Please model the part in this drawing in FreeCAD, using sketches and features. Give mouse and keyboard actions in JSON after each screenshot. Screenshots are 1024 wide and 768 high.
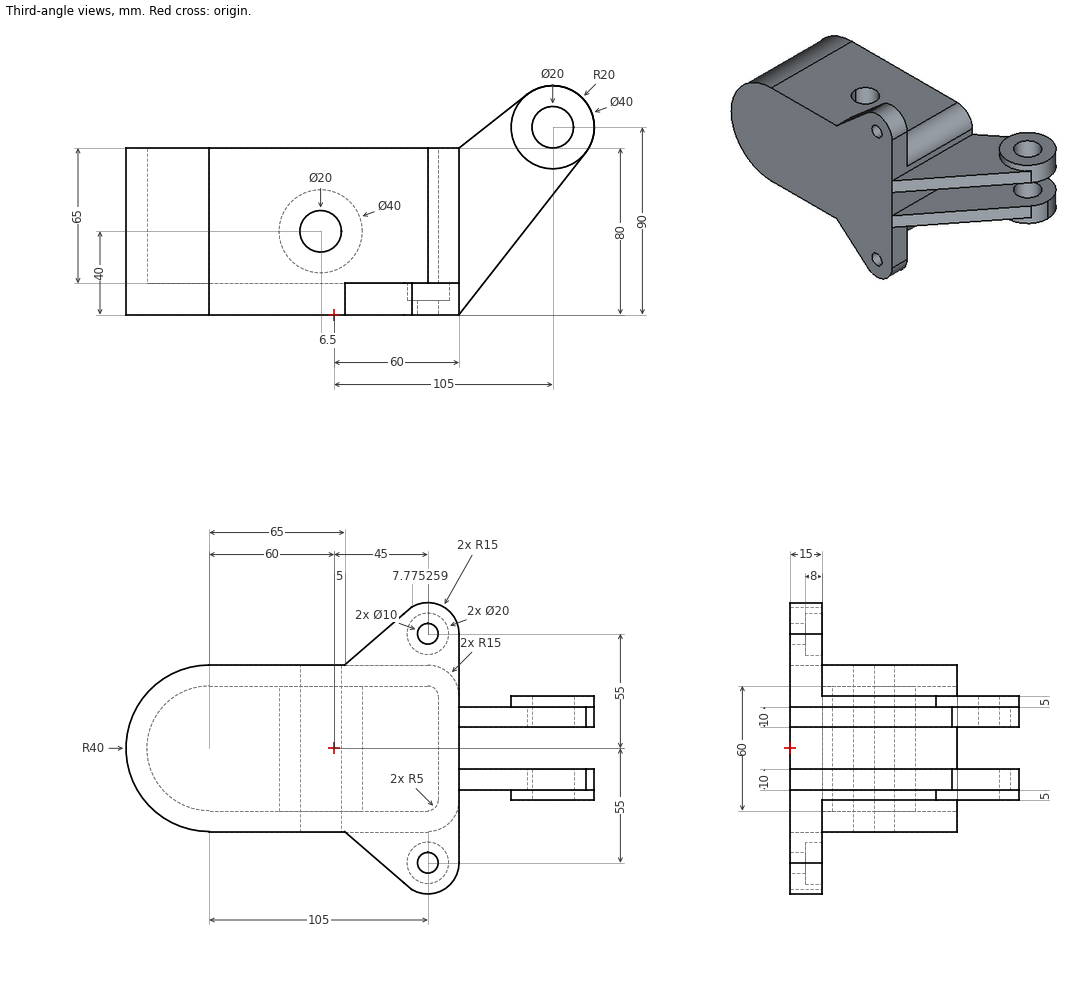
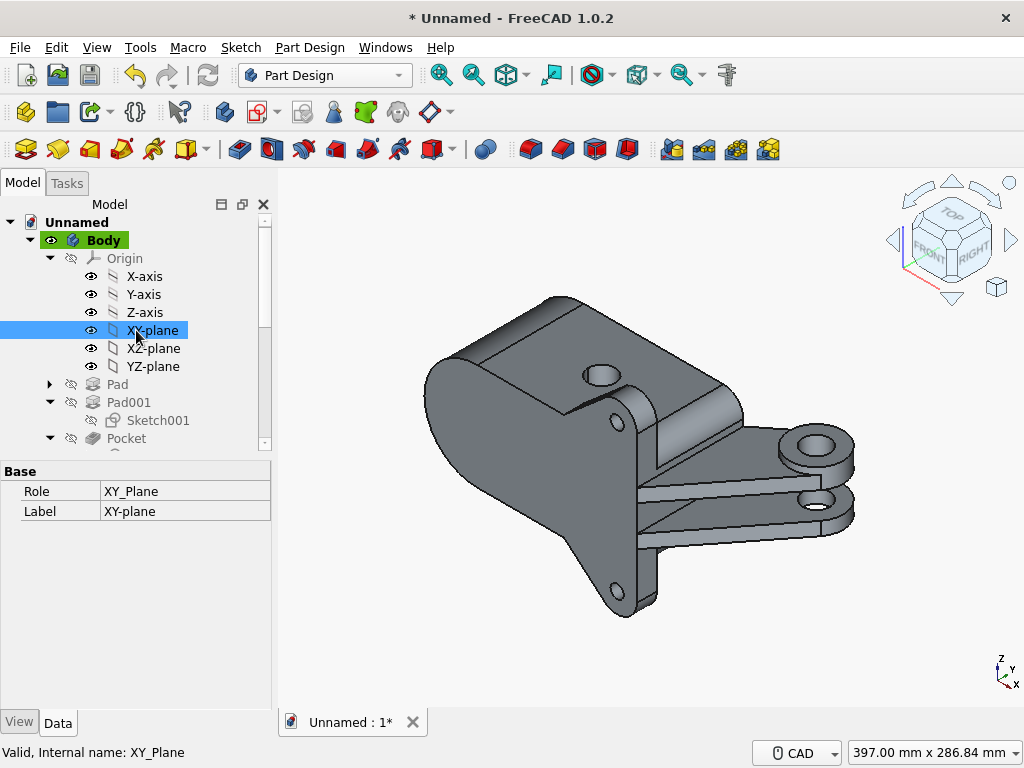
{"action": "left_click", "coordinate": [430, 112]}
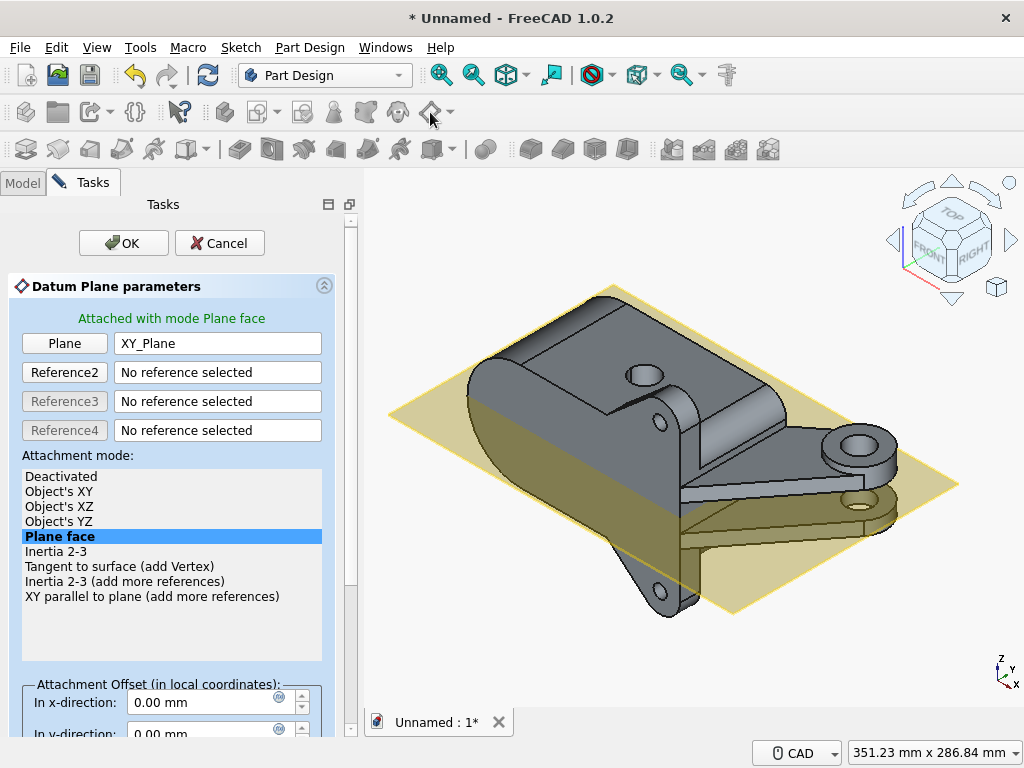
{"action": "scroll", "coordinate": [351, 475], "scroll_direction": "down", "scroll_amount": 2}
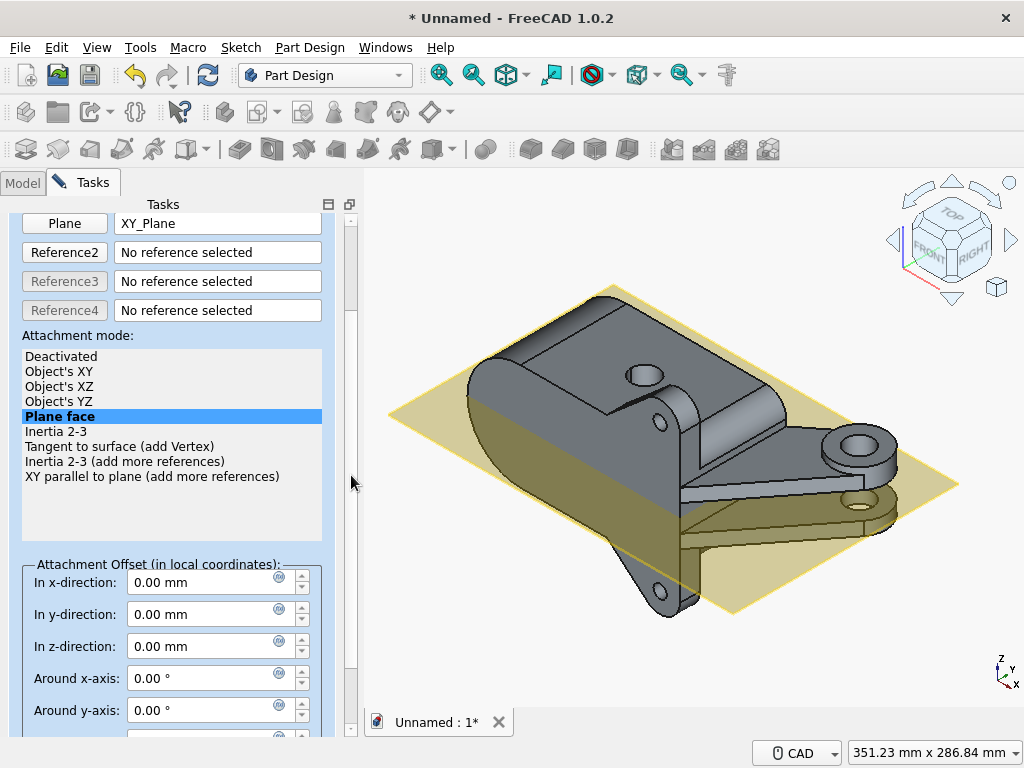
{"action": "triple_click", "coordinate": [210, 646]}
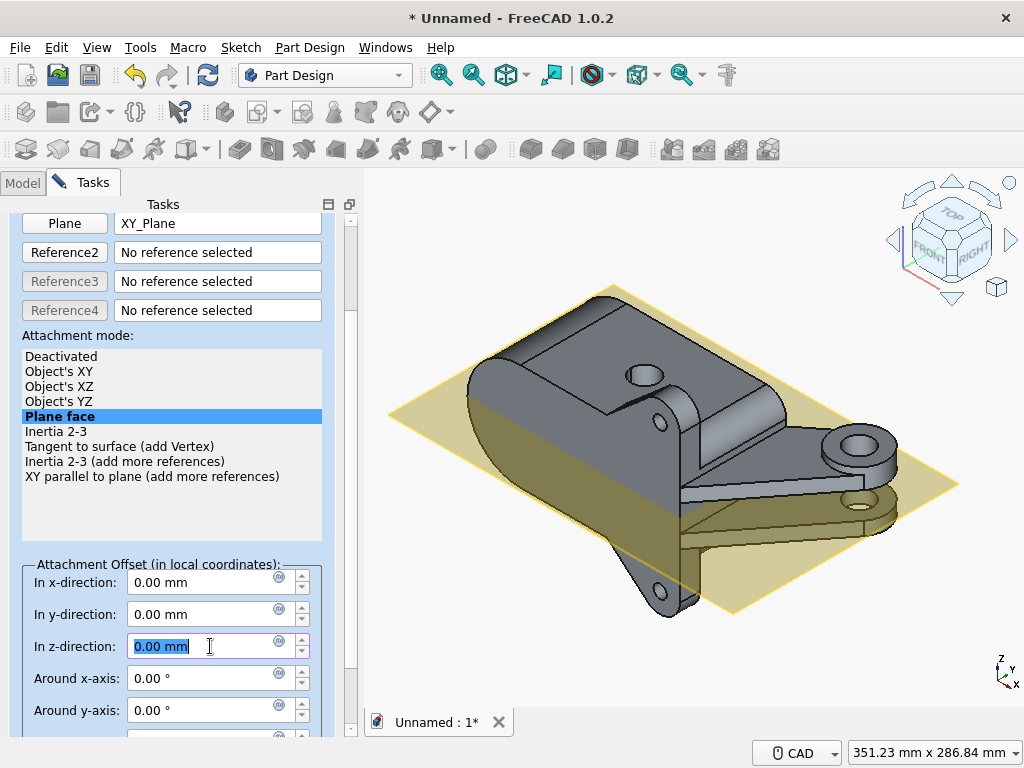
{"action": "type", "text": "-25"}
{"action": "key", "text": "Tab"}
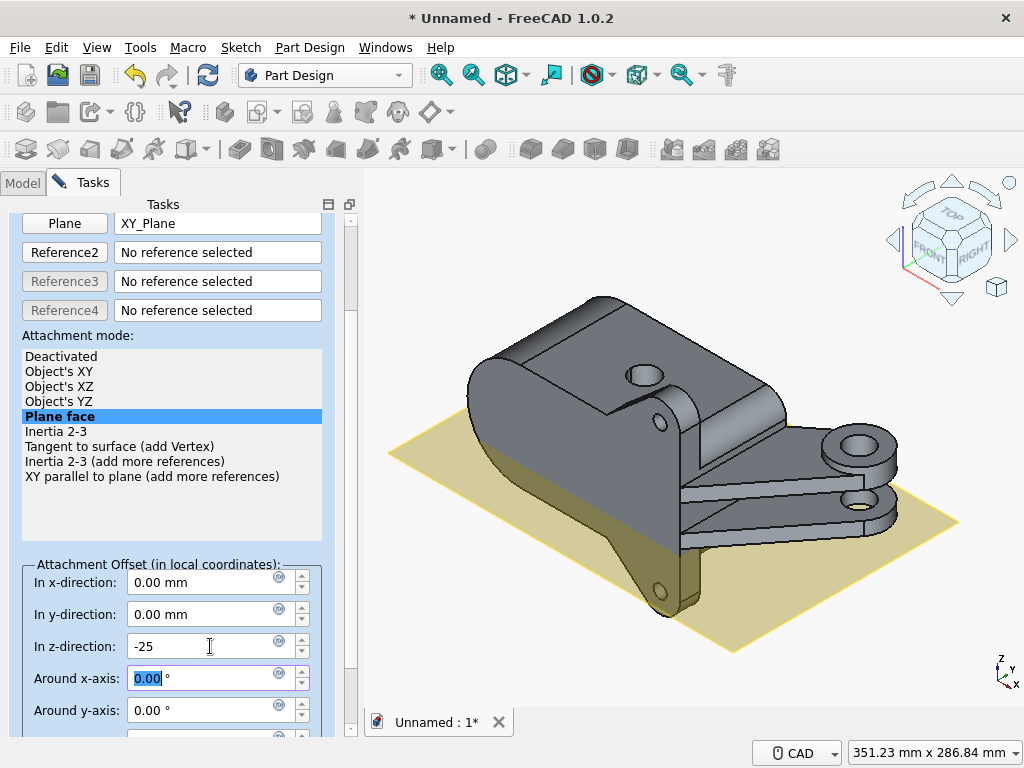
{"action": "scroll", "coordinate": [351, 475], "scroll_direction": "up", "scroll_amount": 3}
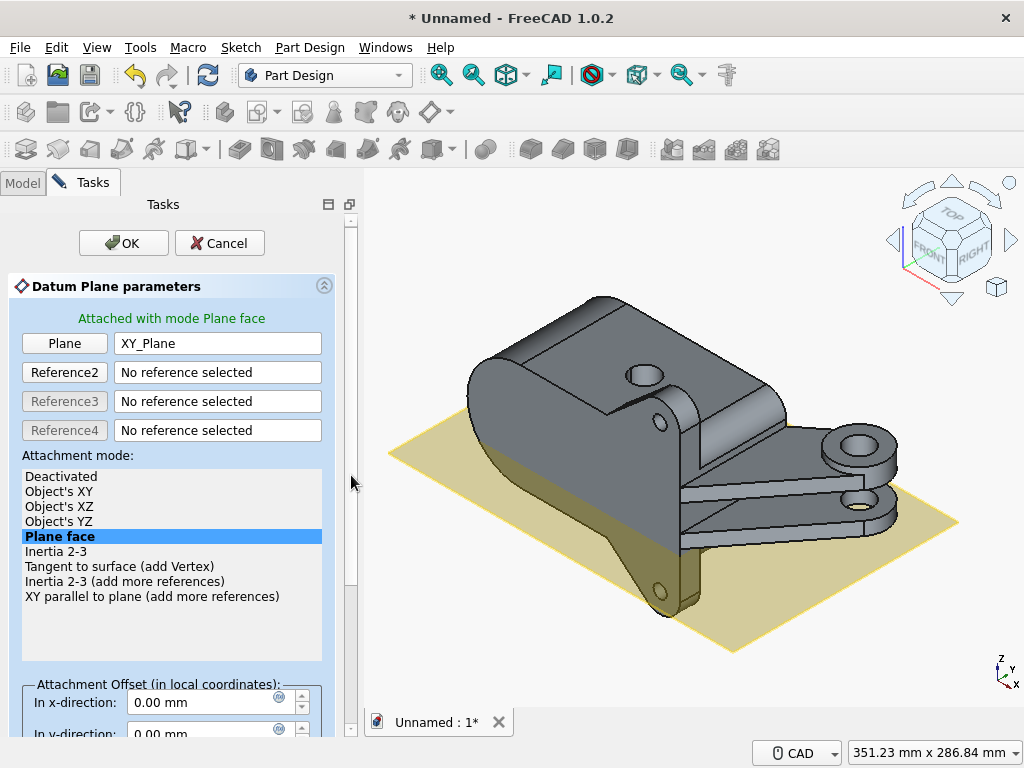
{"action": "left_click", "coordinate": [124, 243]}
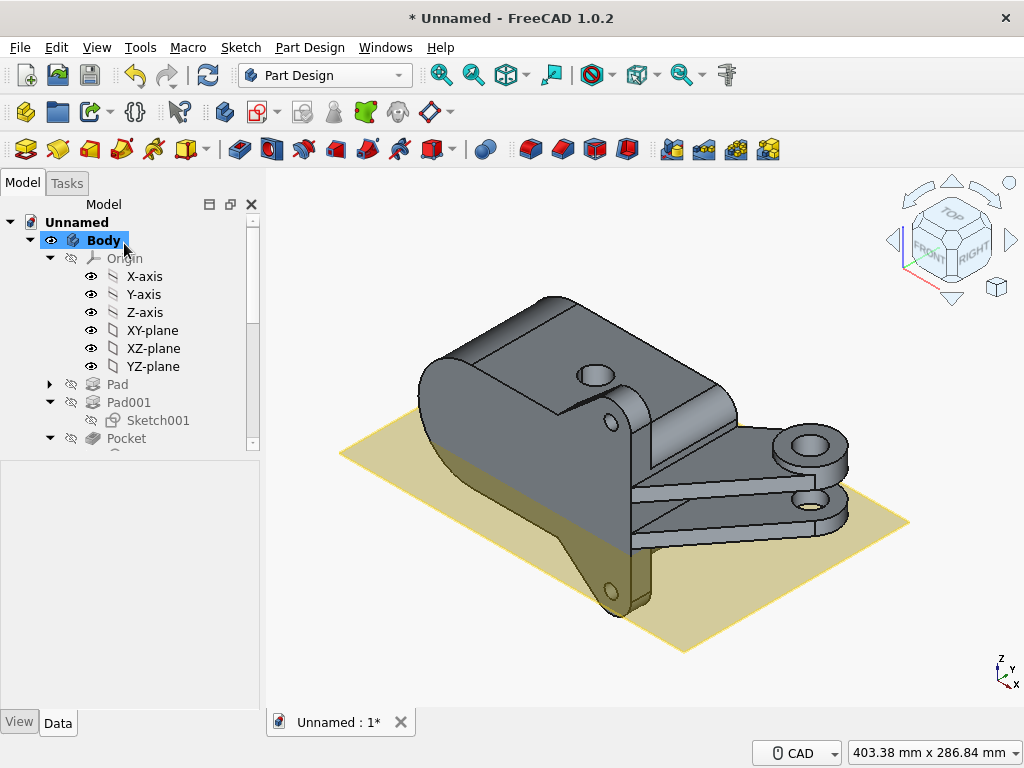
{"action": "scroll", "coordinate": [100, 326], "scroll_direction": "down", "scroll_amount": 3}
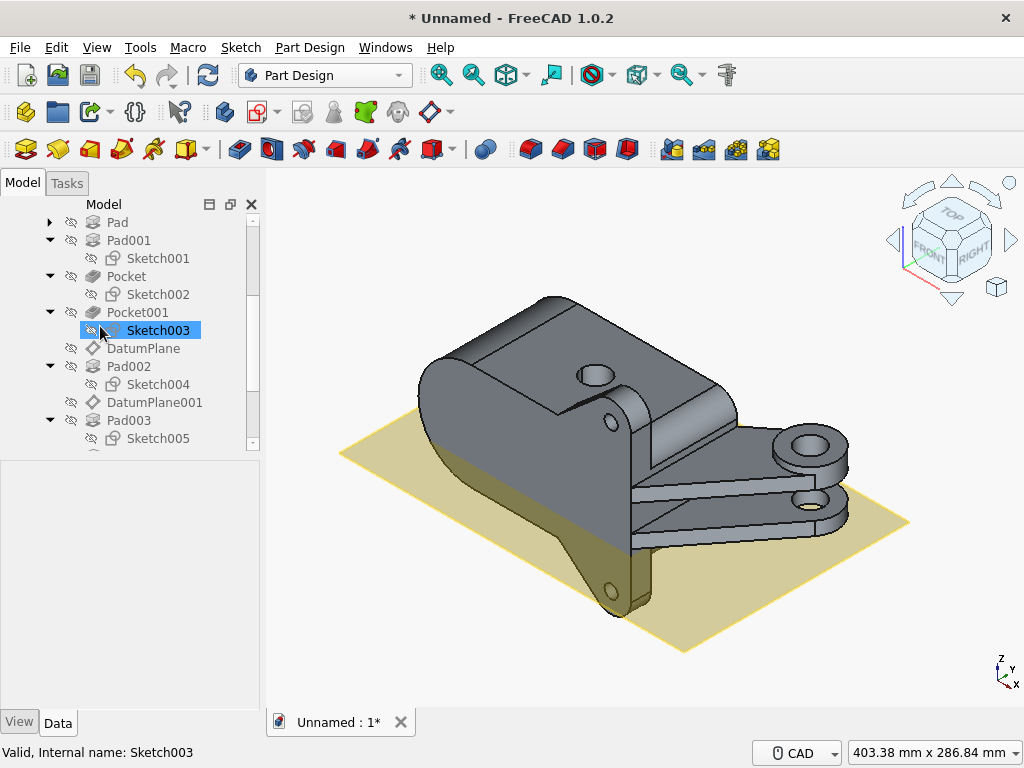
{"action": "scroll", "coordinate": [140, 326], "scroll_direction": "up", "scroll_amount": 15}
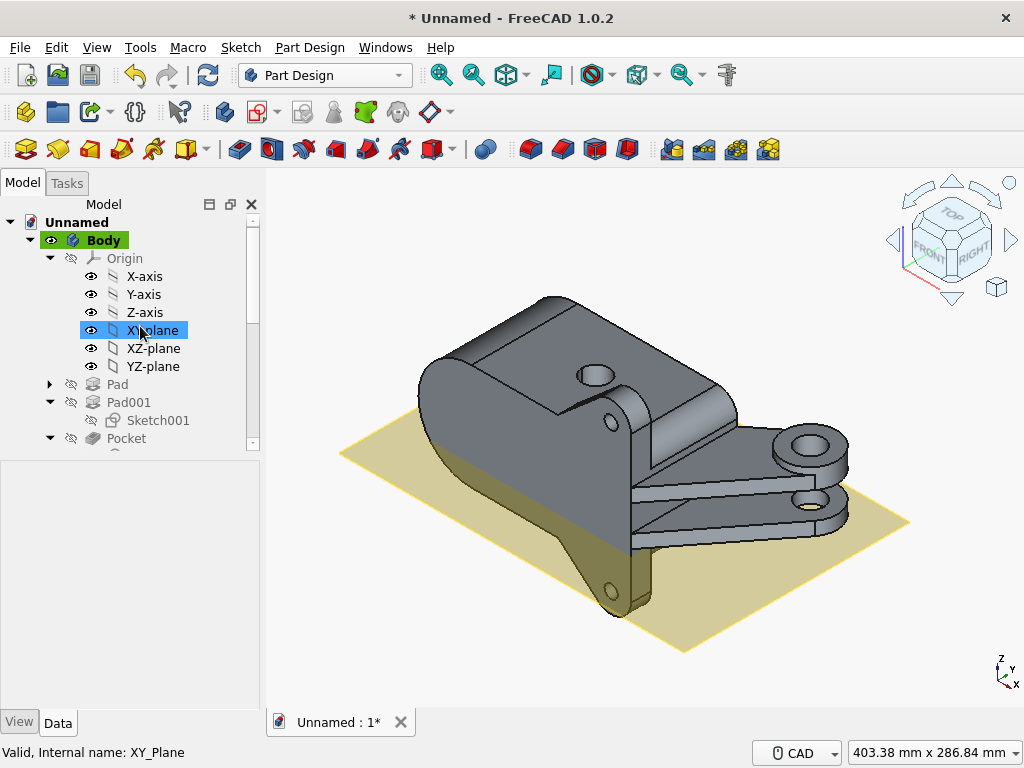
{"action": "scroll", "coordinate": [100, 326], "scroll_direction": "down", "scroll_amount": 6}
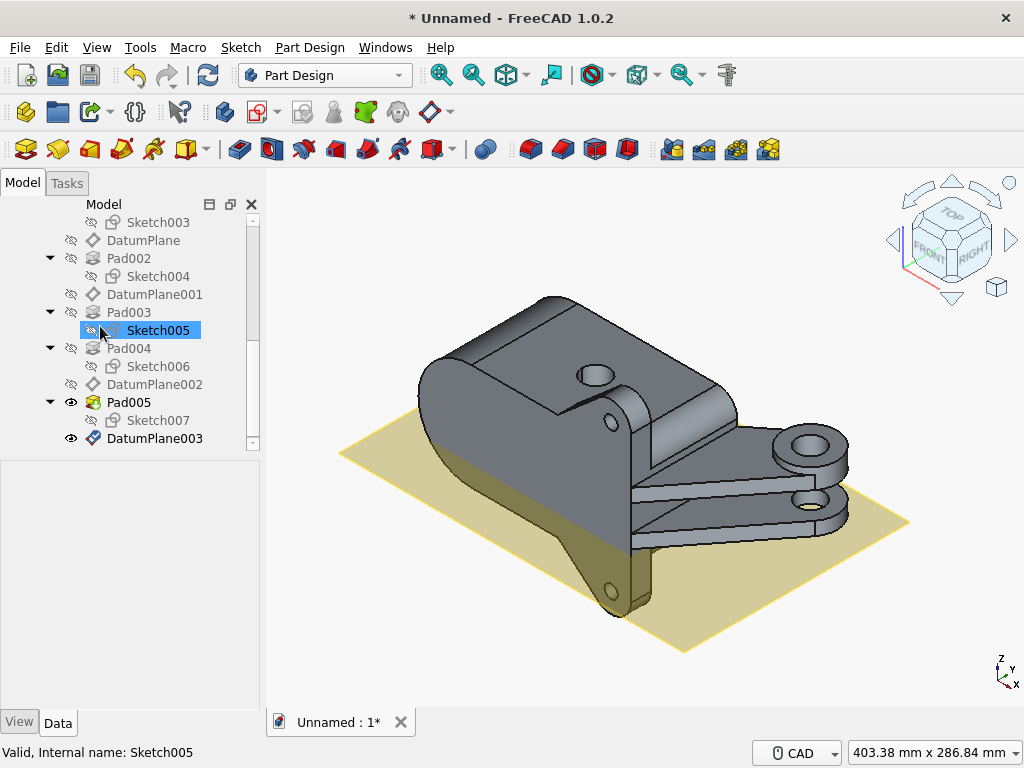
{"action": "left_click", "coordinate": [116, 438]}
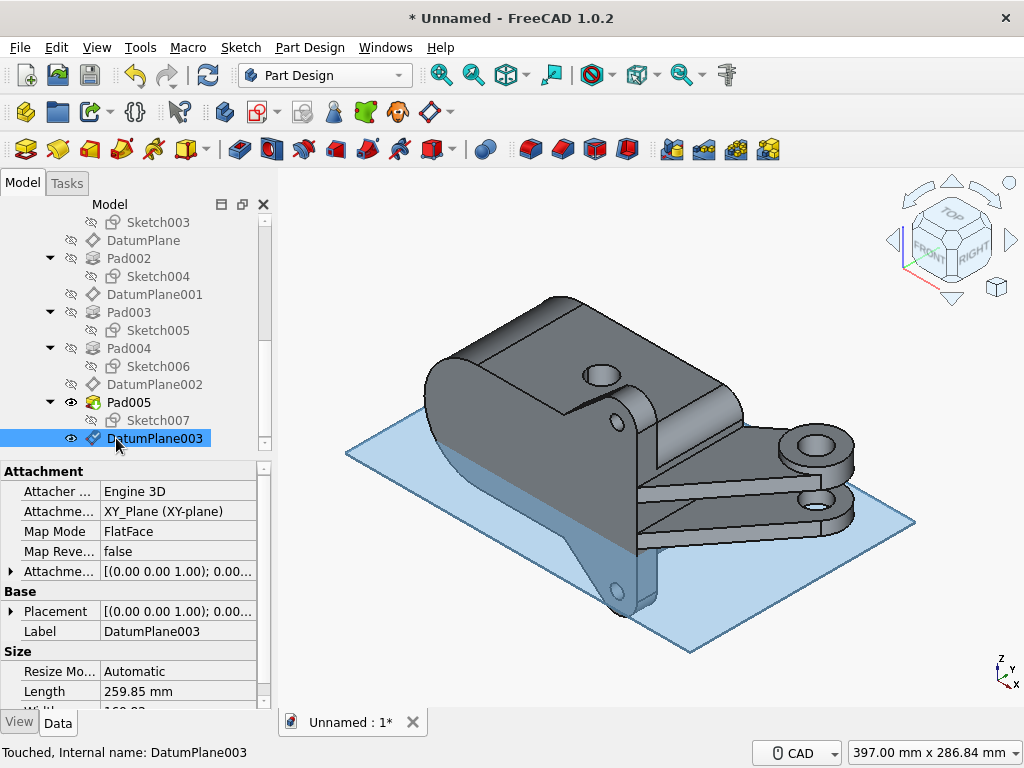
{"action": "left_click", "coordinate": [258, 112]}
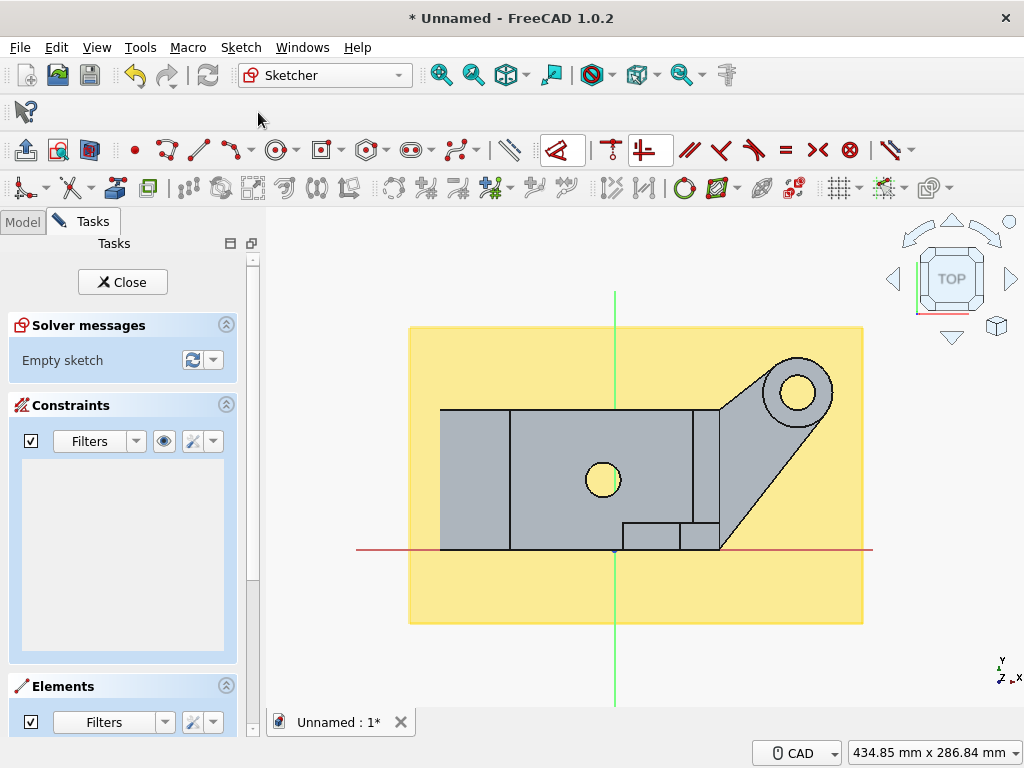
{"action": "left_click", "coordinate": [90, 150]}